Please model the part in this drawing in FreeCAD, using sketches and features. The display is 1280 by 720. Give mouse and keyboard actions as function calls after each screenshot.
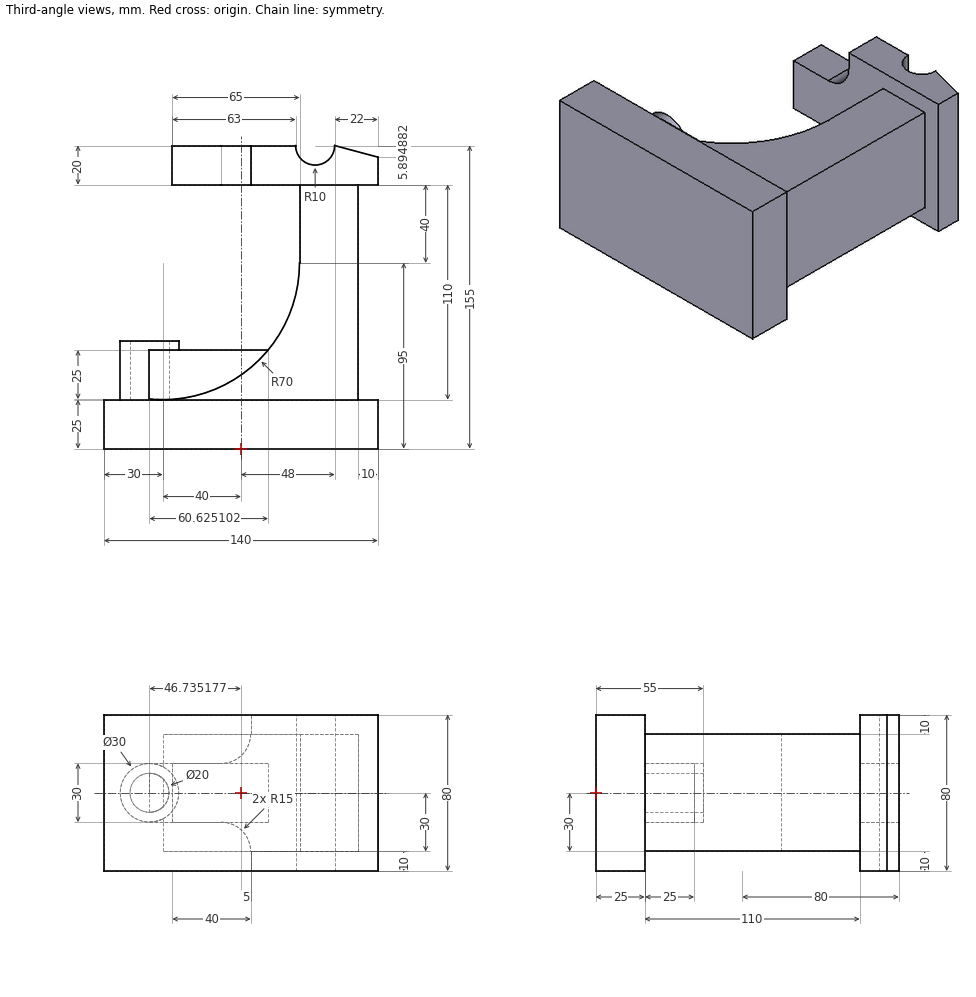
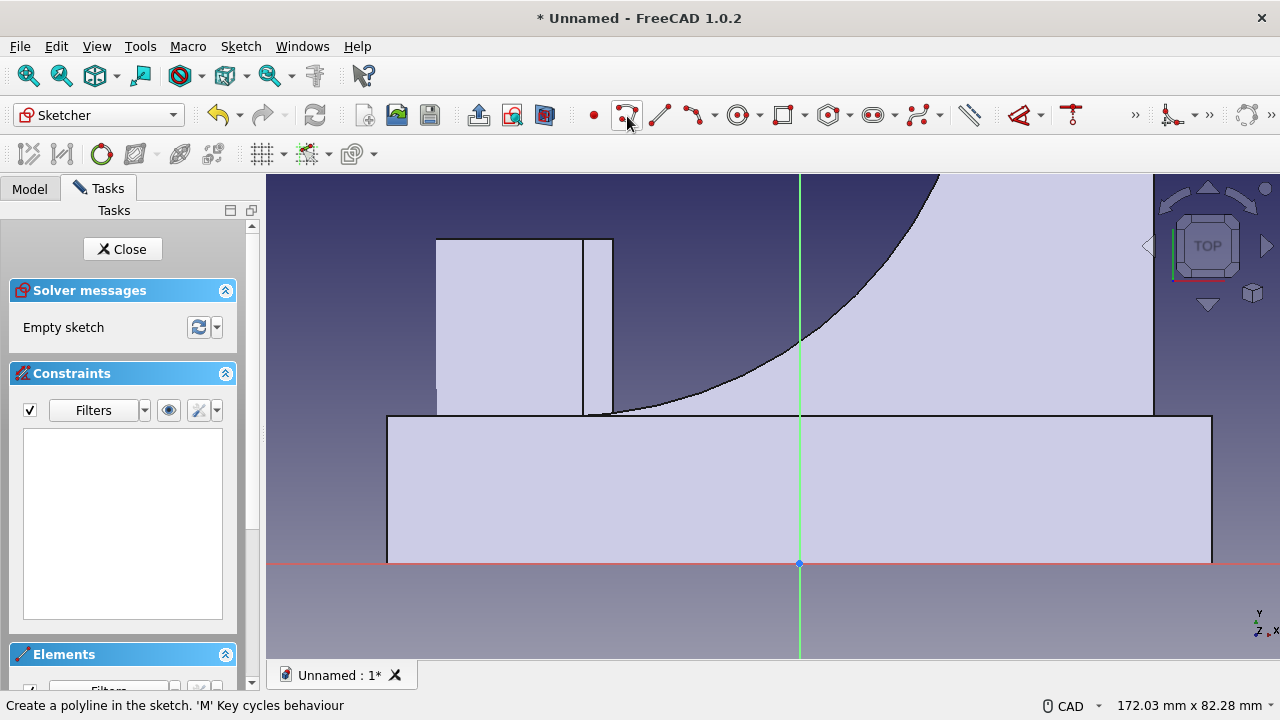
click(882, 267)
click(524, 267)
click(524, 414)
right_click(524, 414)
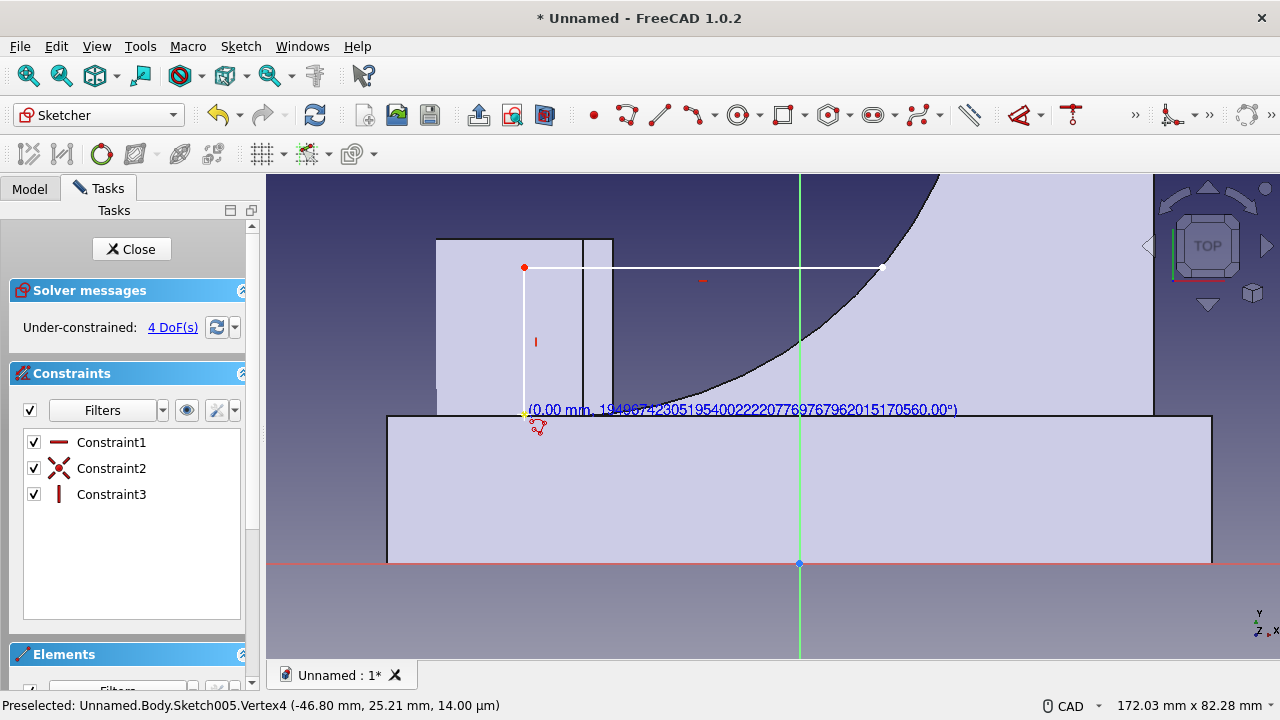
click(692, 116)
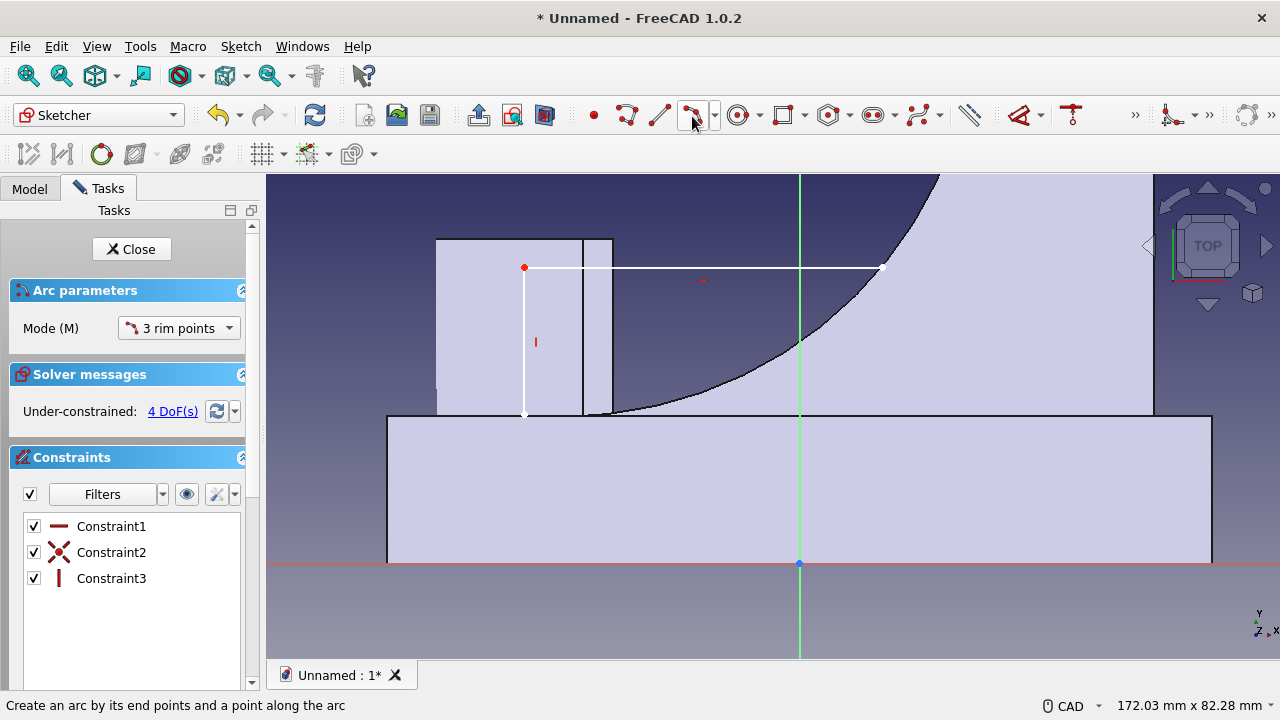
click(524, 415)
click(882, 268)
click(721, 385)
key(Escape)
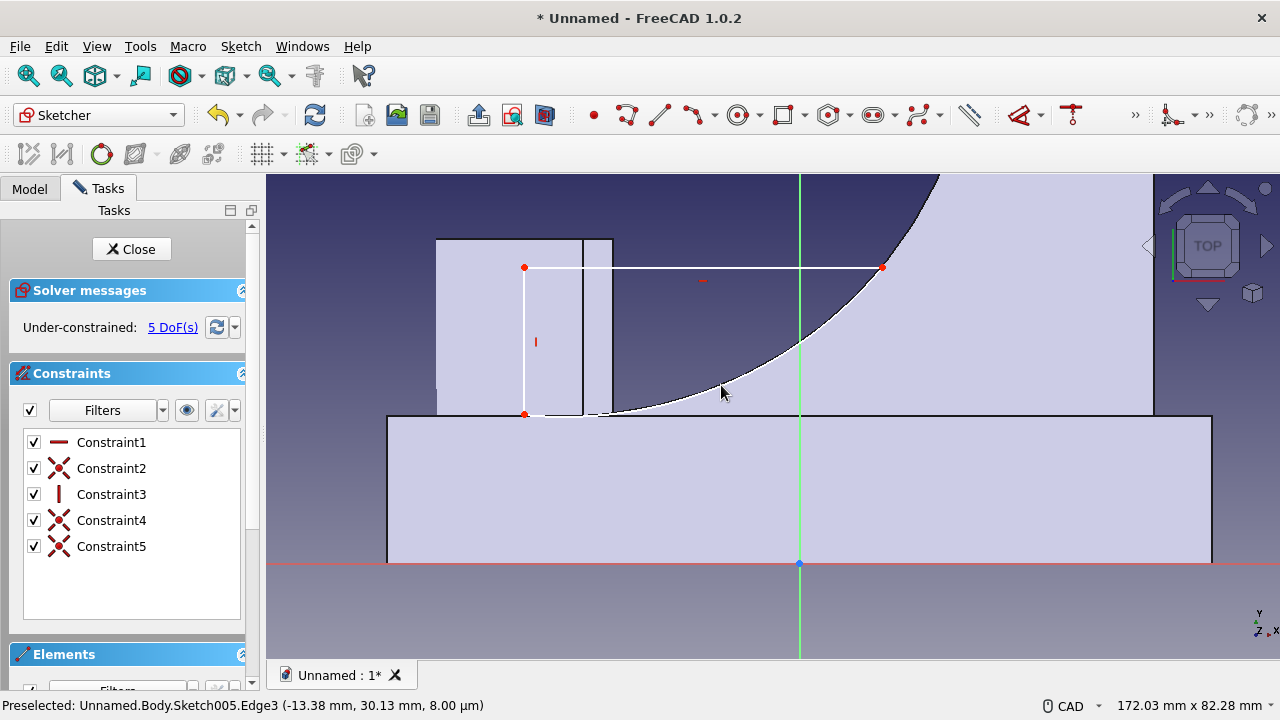
click(1018, 116)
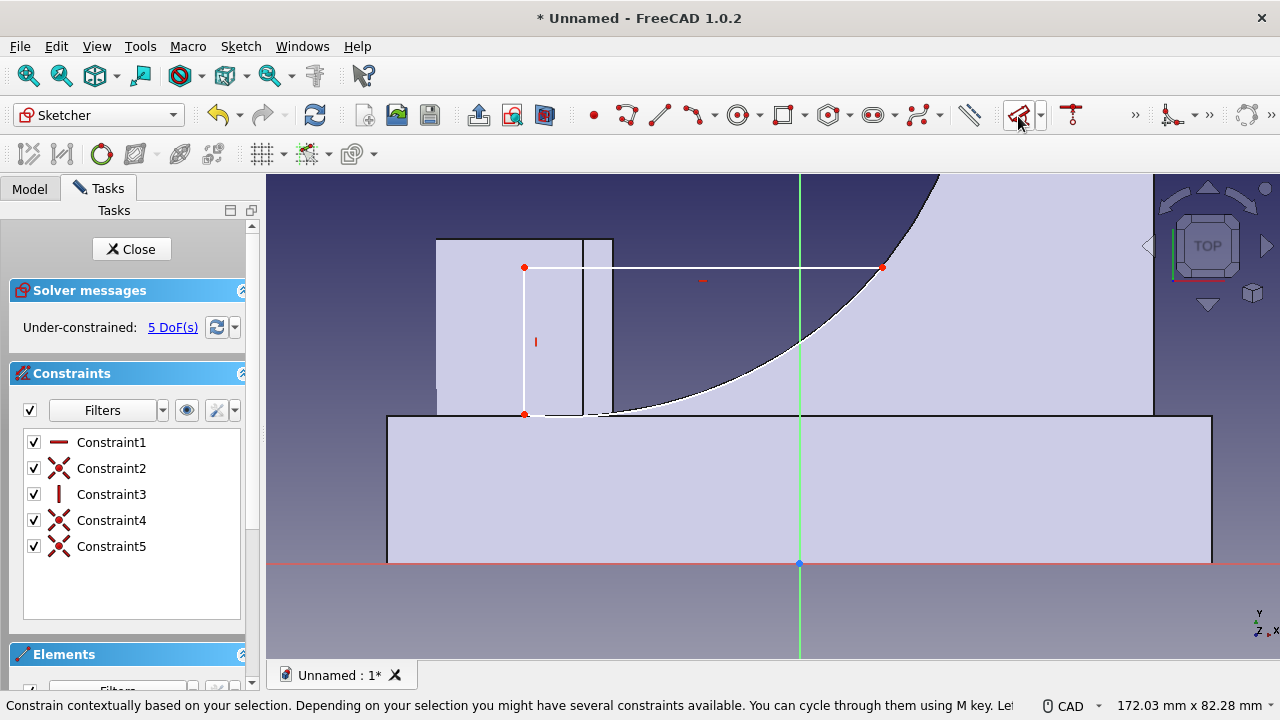
click(644, 409)
click(650, 440)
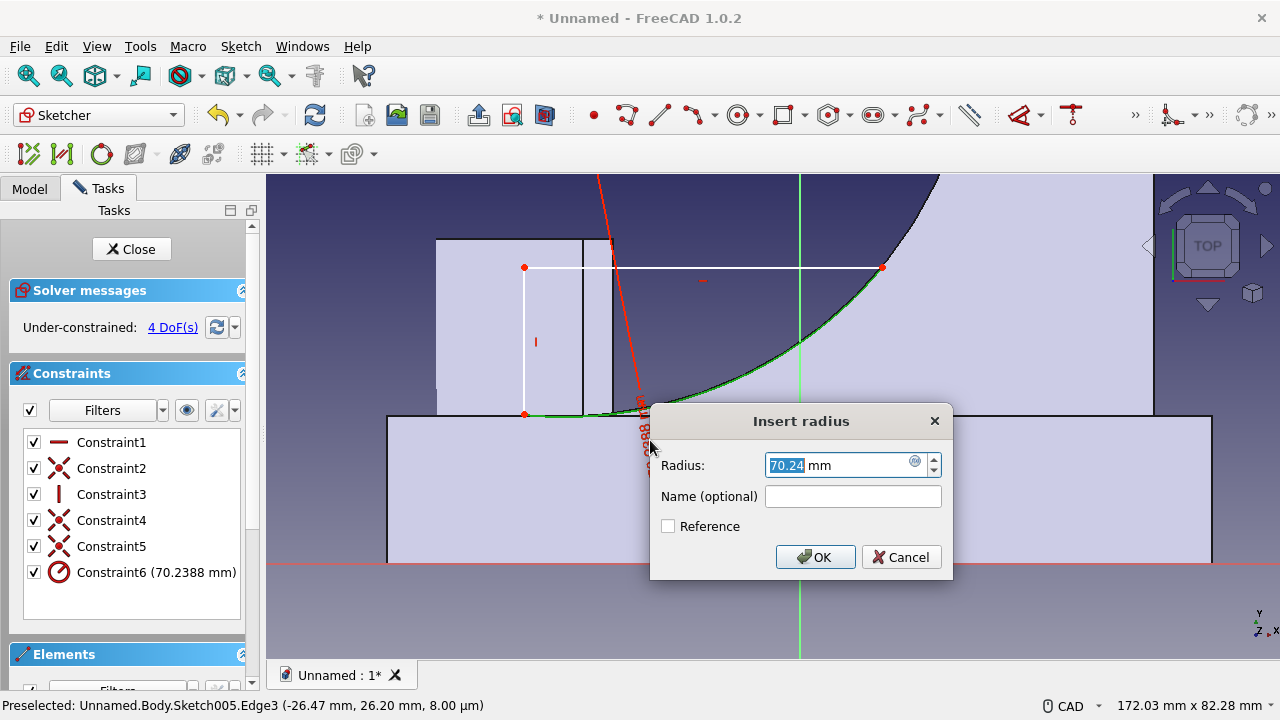
text(70)
key(Return)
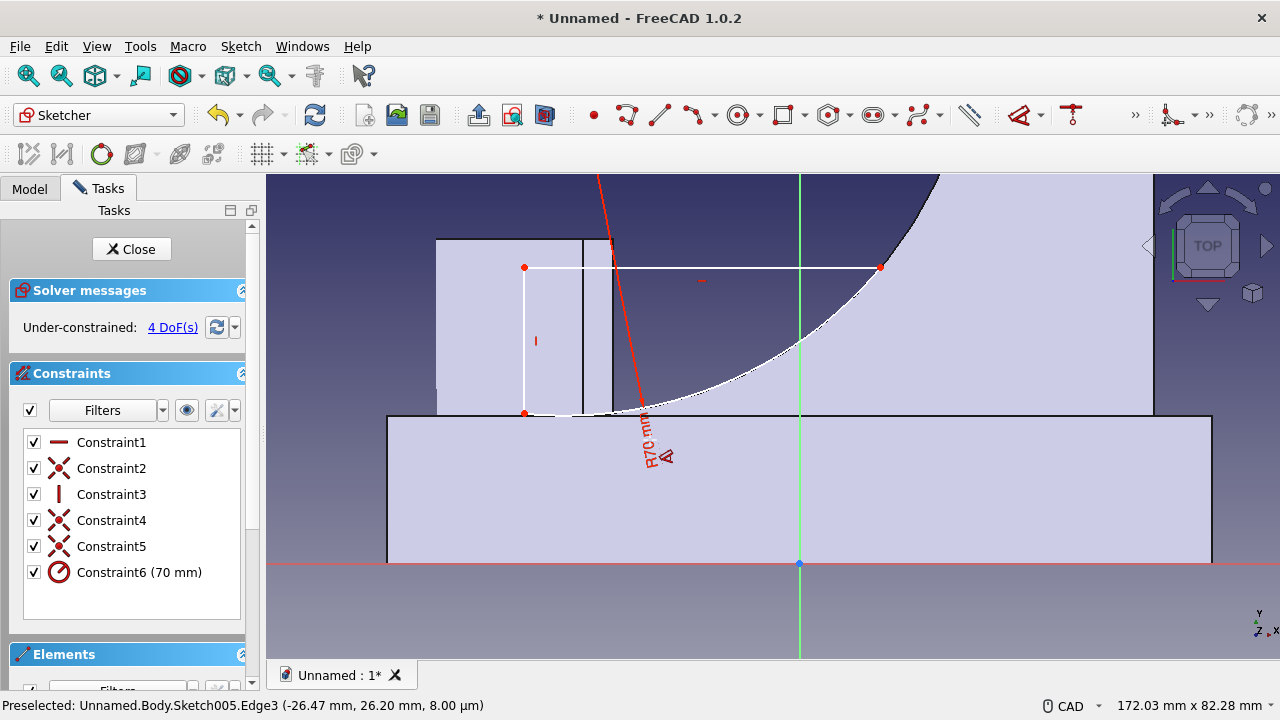
click(524, 312)
click(490, 341)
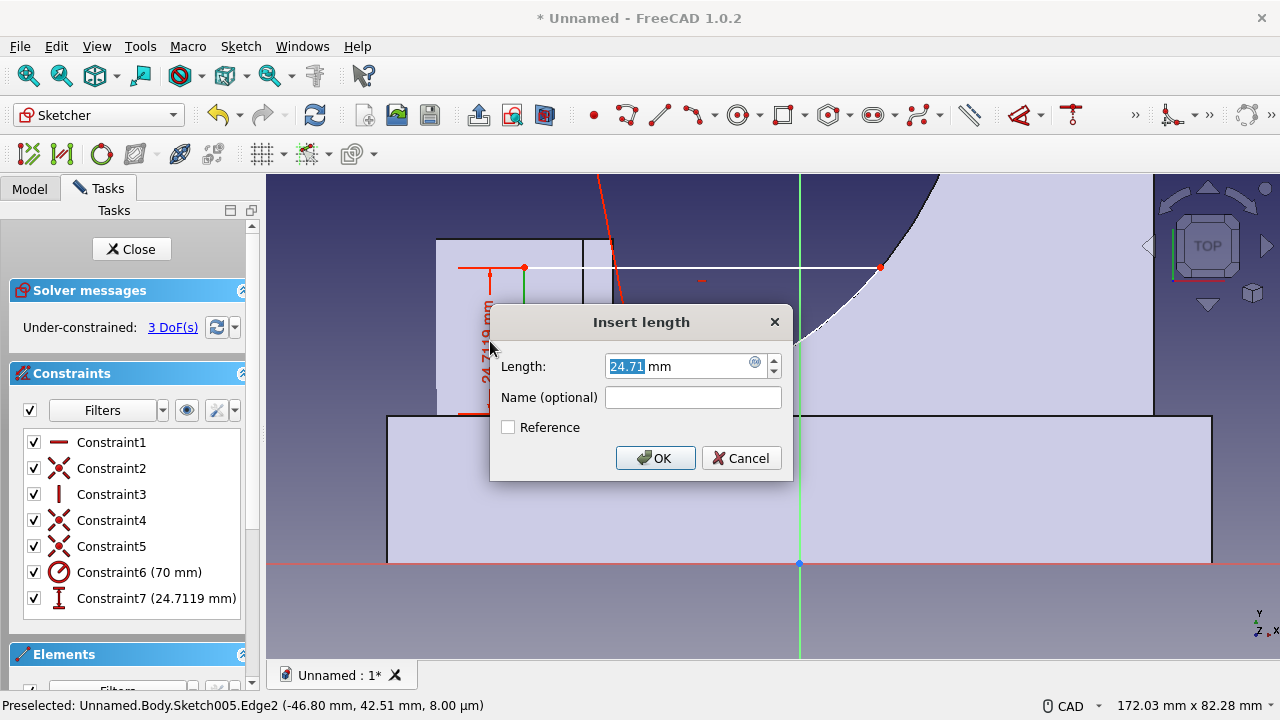
text(25)
key(Return)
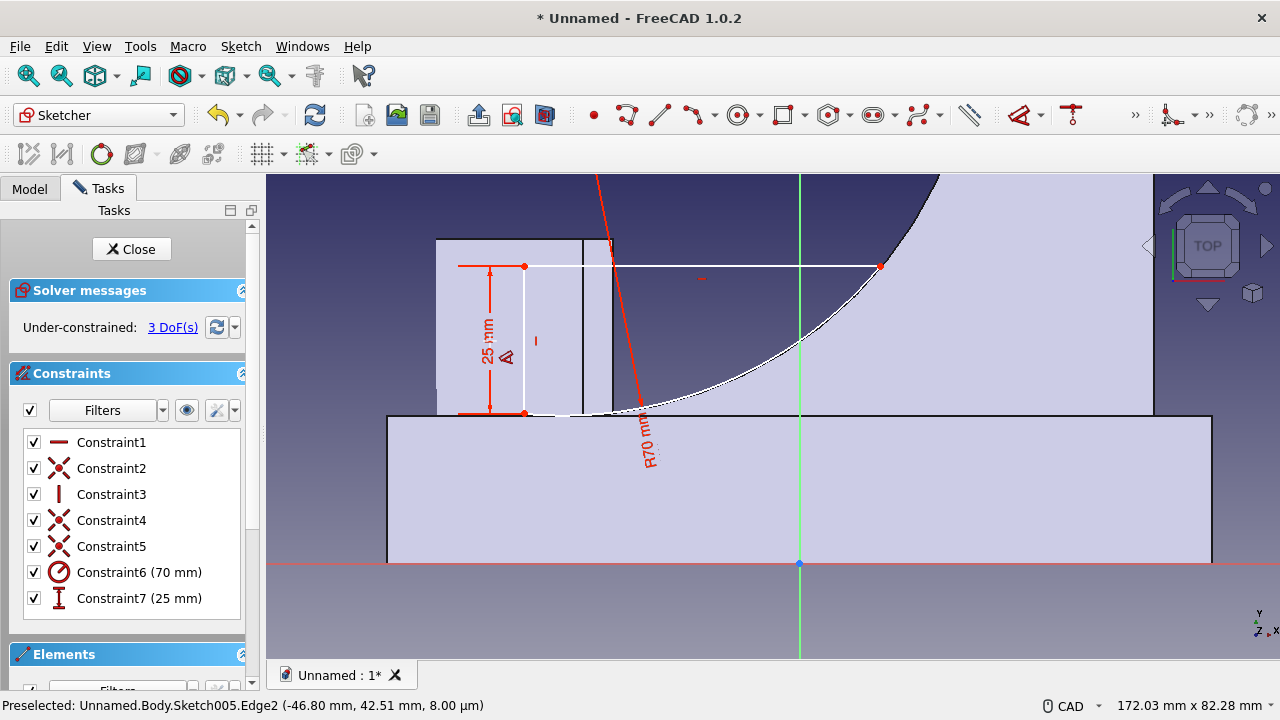
scroll(706, 579, down, 3)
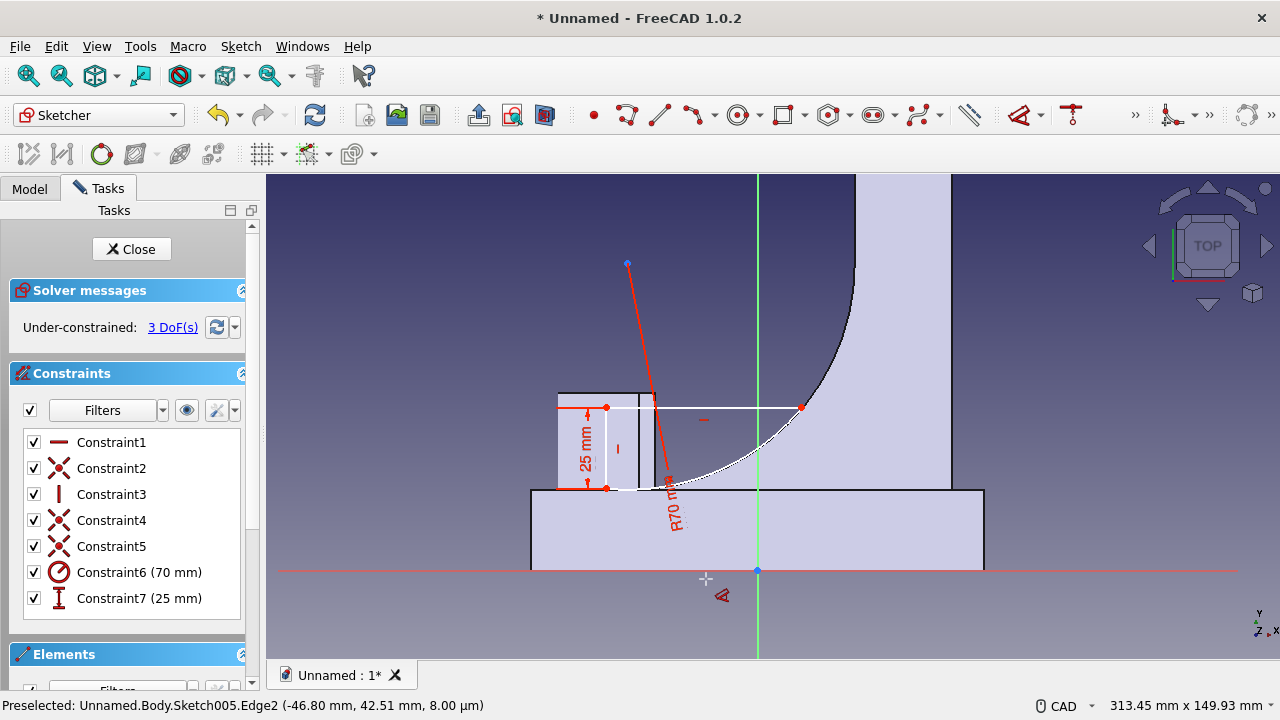
click(628, 263)
click(693, 229)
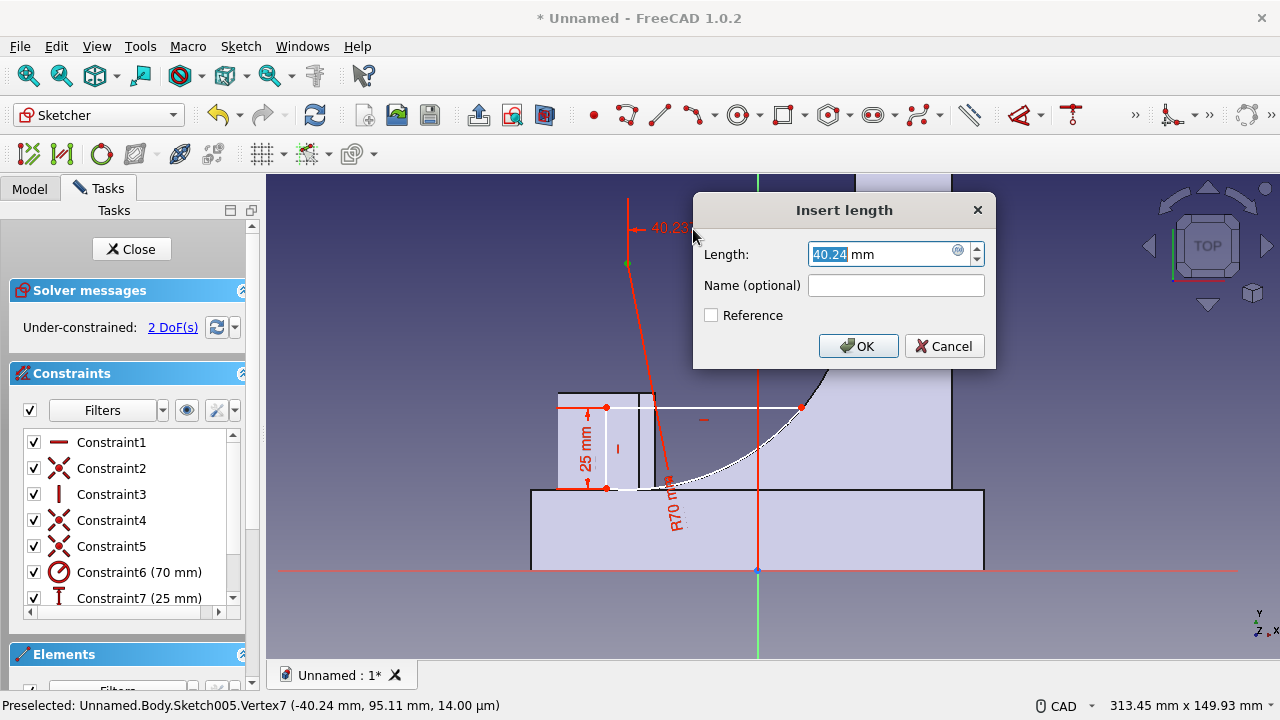
text(40)
key(Return)